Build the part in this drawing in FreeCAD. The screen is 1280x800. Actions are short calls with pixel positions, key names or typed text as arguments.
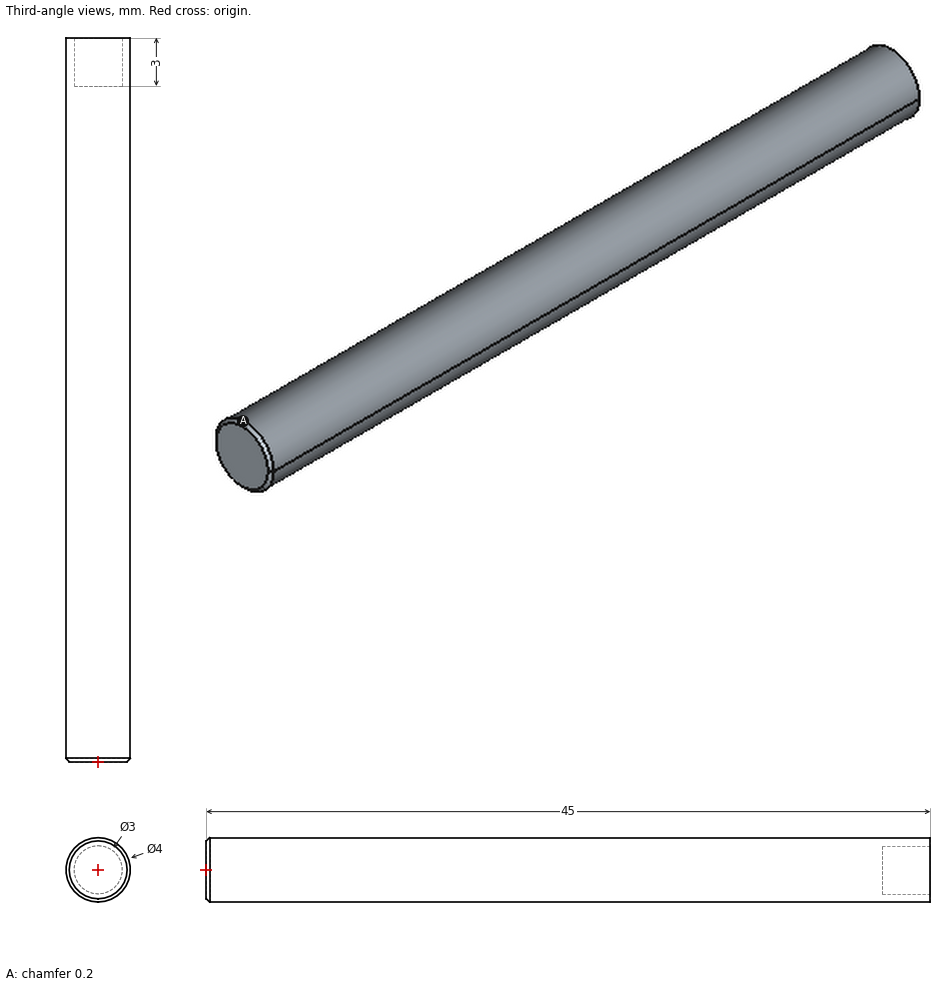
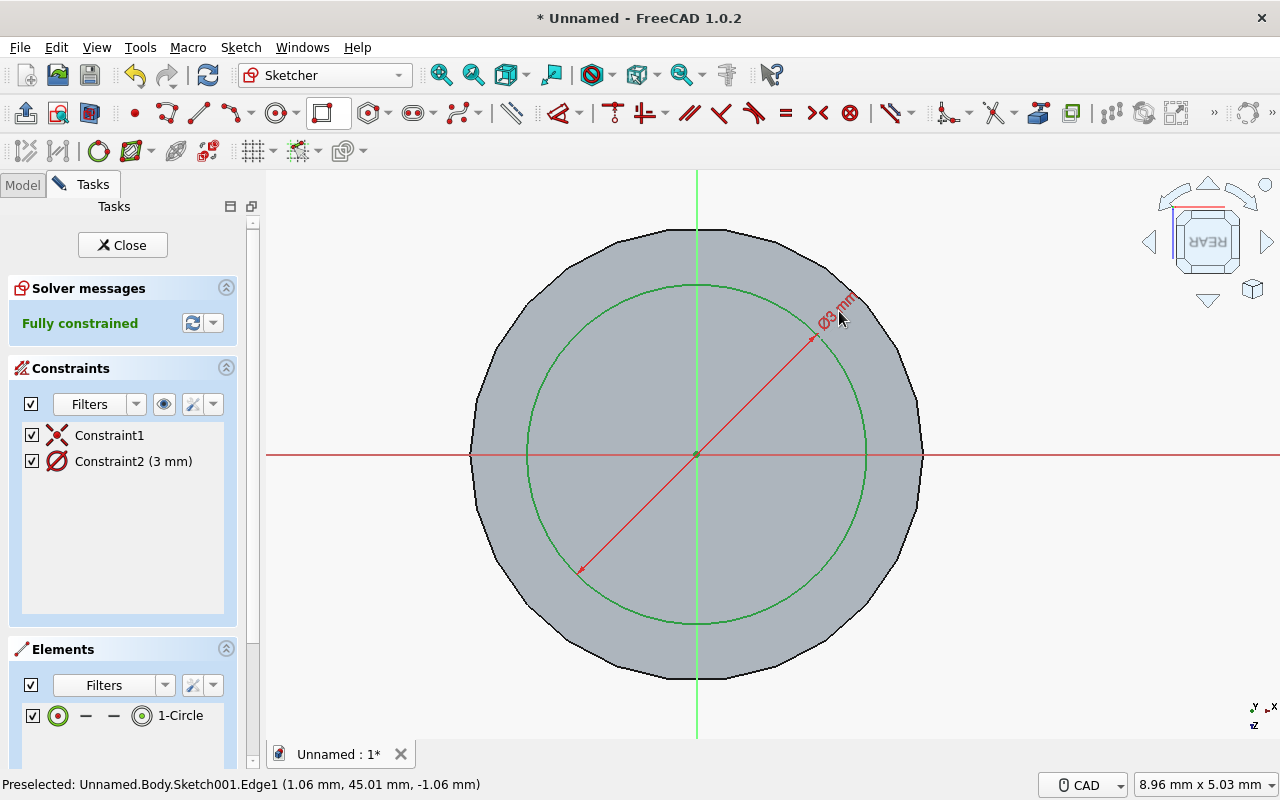
click(123, 245)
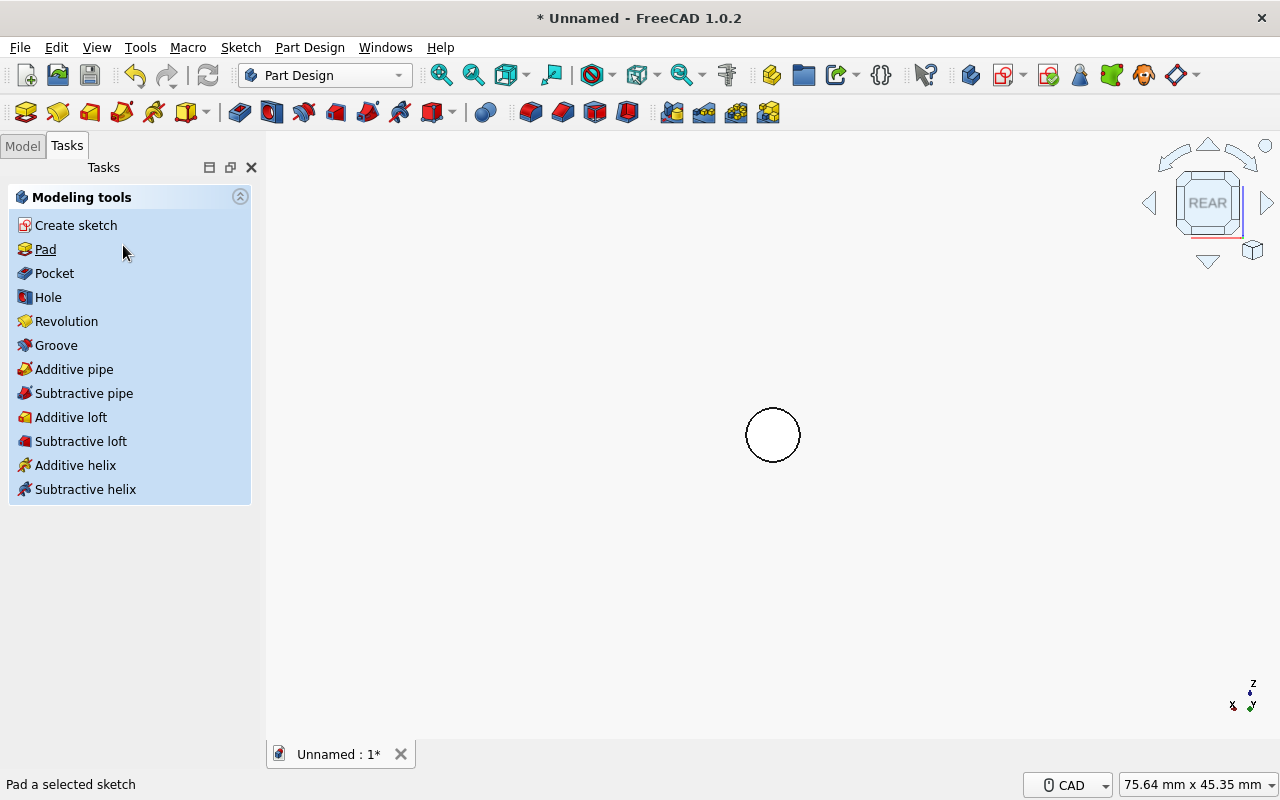
click(240, 112)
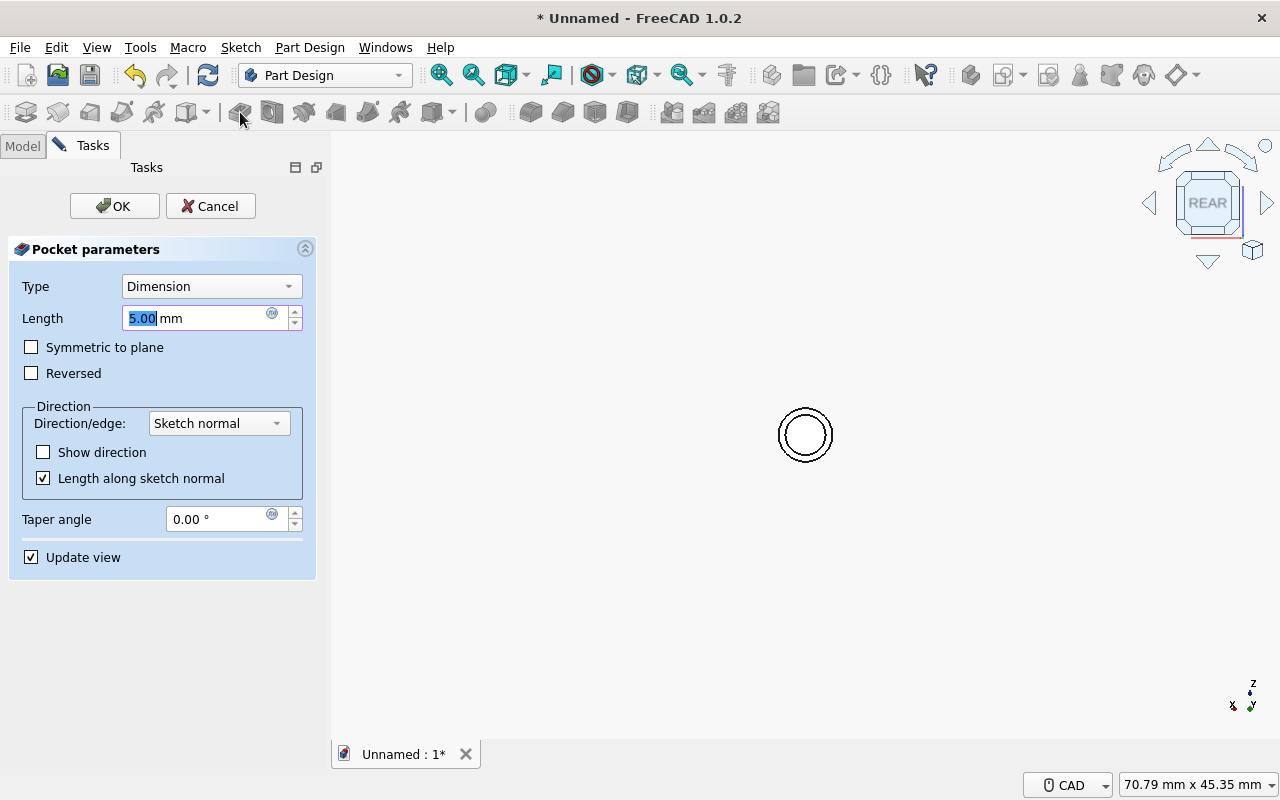
text(3)
key(Tab)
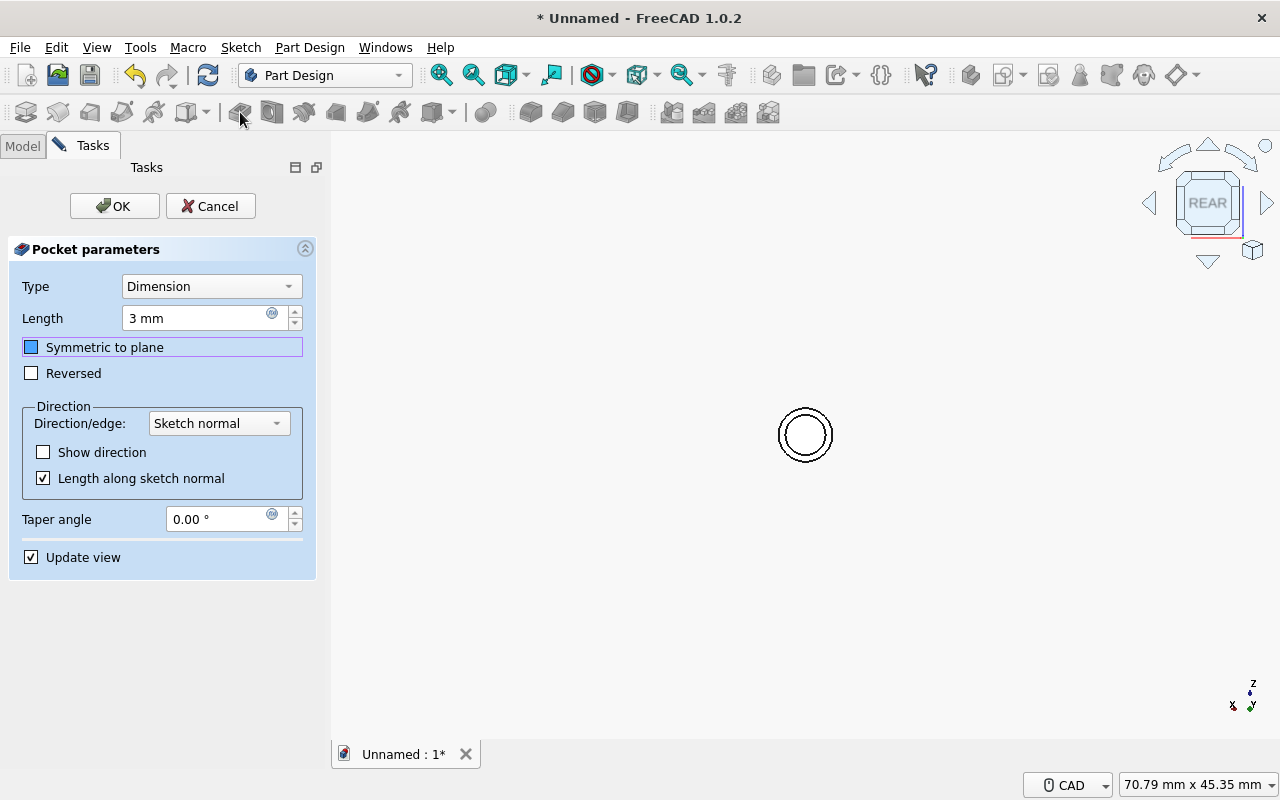
click(115, 206)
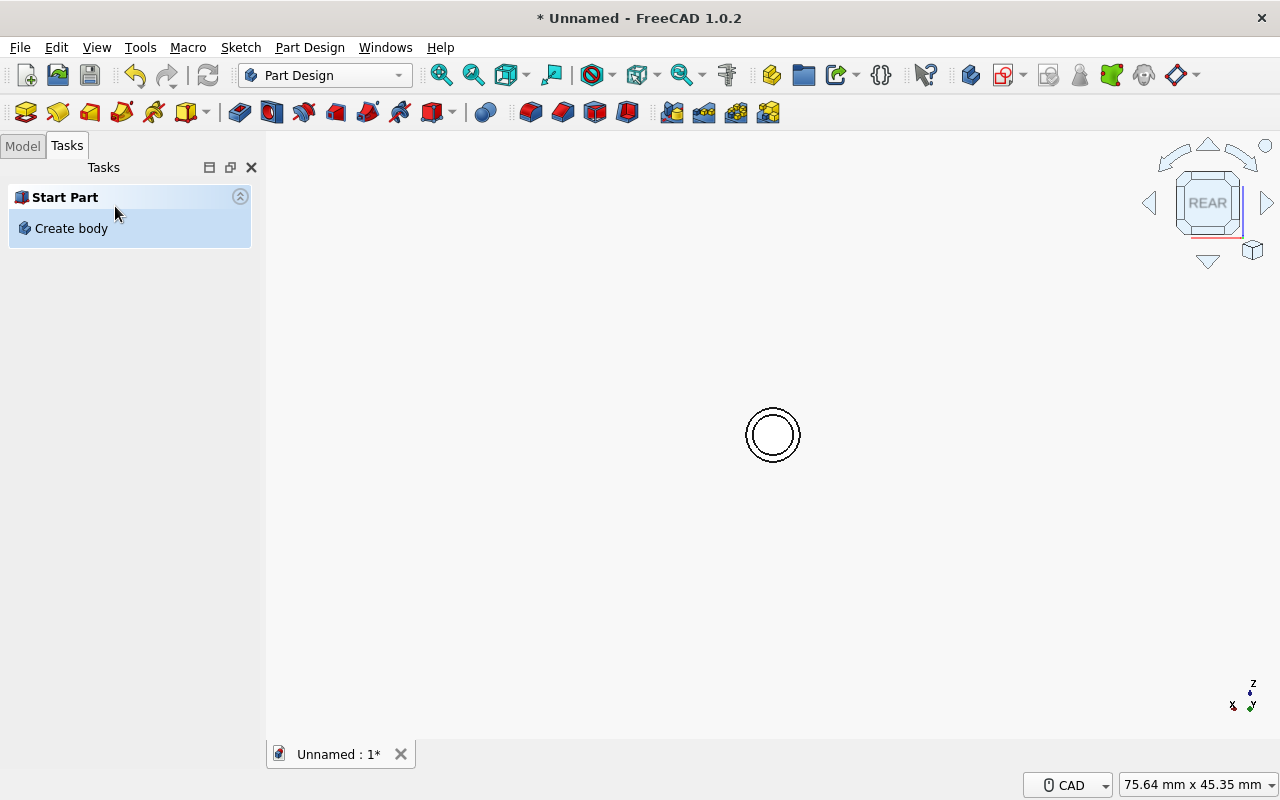
key(0)